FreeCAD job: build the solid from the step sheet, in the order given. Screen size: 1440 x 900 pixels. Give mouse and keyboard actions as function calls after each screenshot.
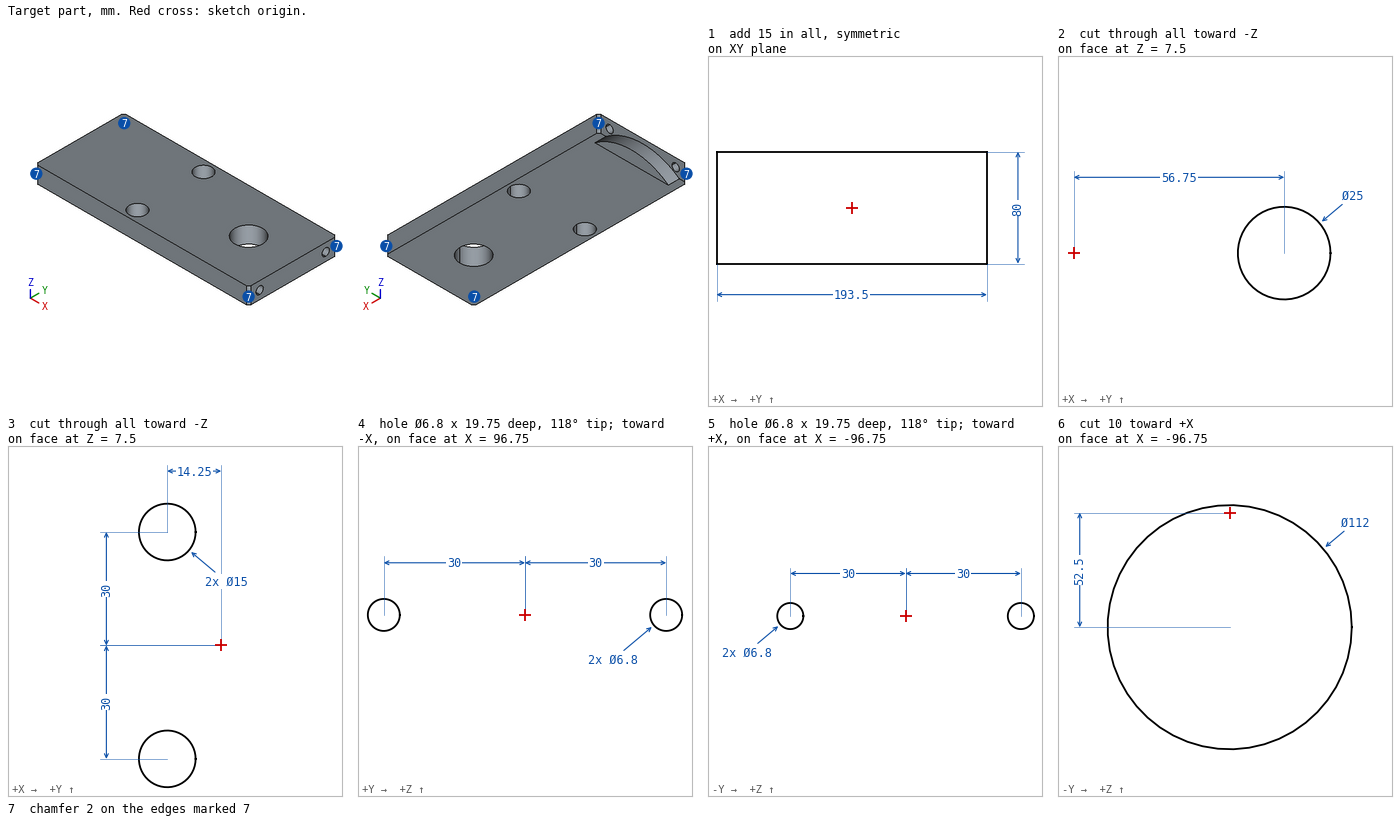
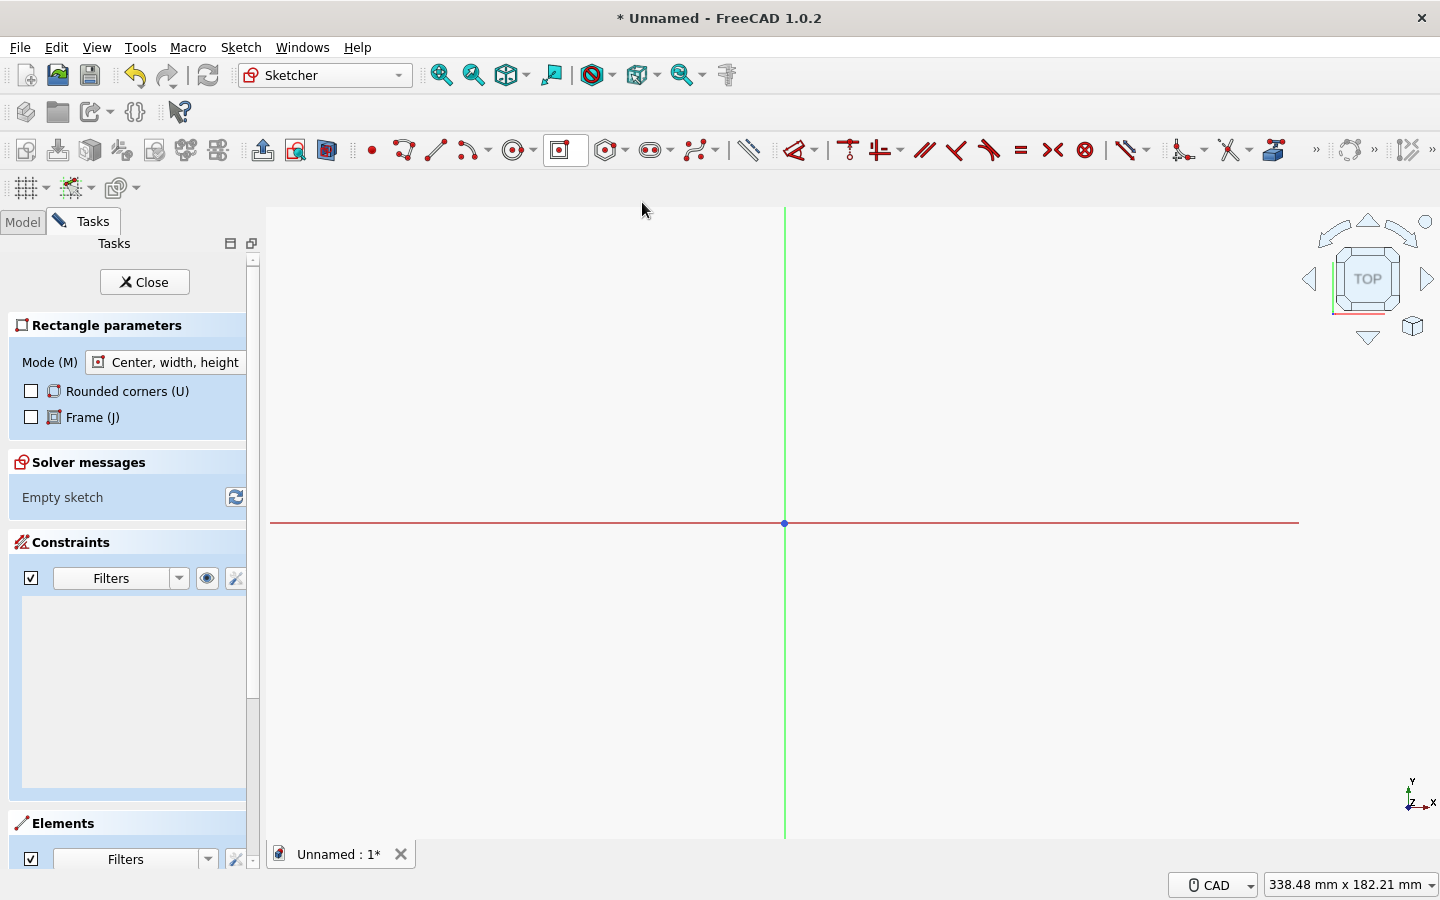
click(785, 523)
move(1120, 384)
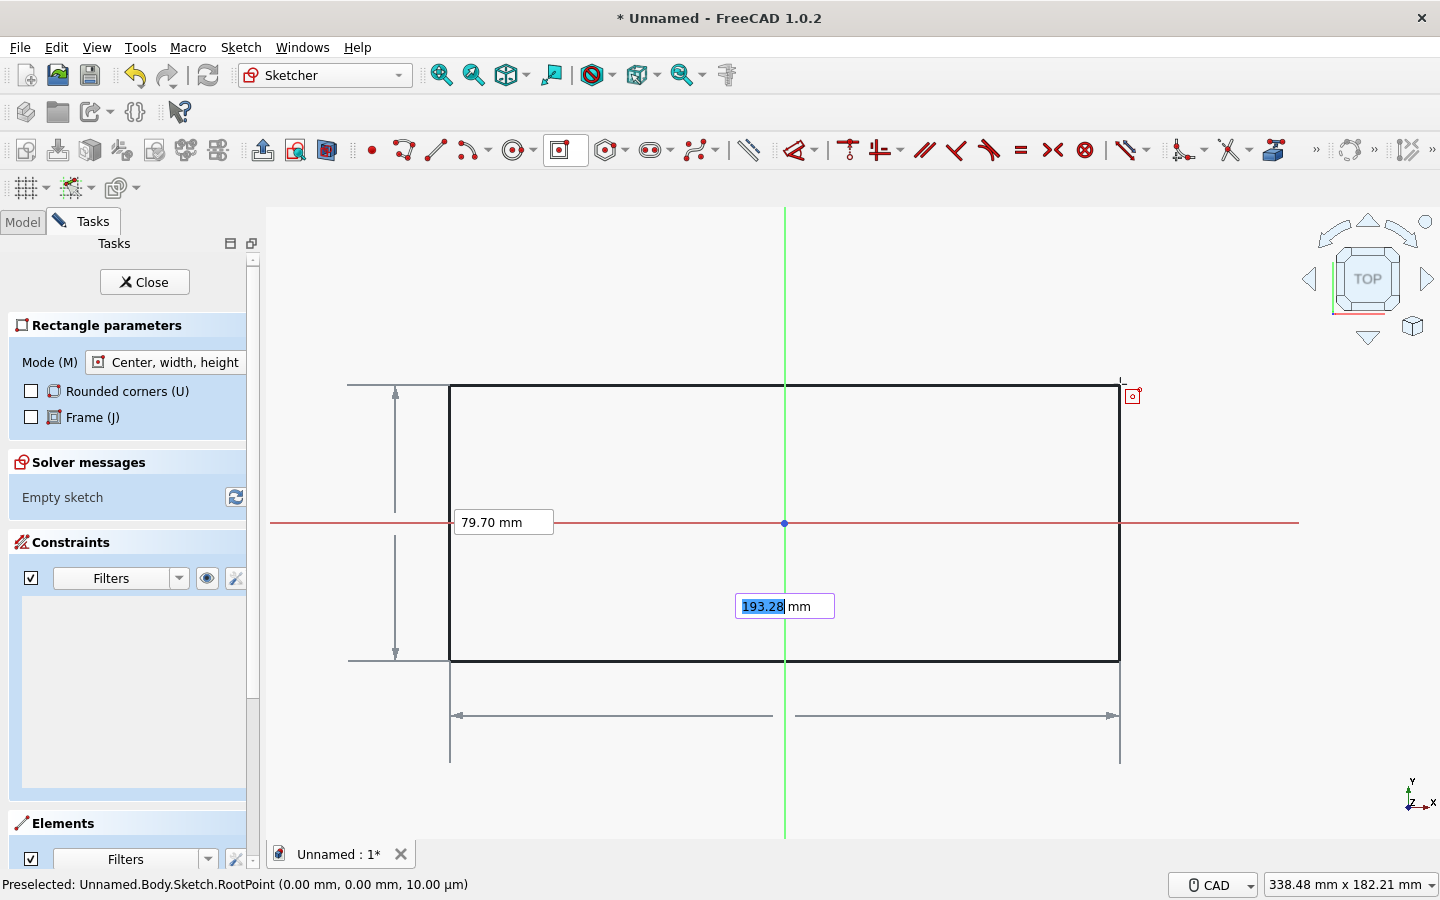
text(193.5)
key(Tab)
text(80)
key(Return)
key(Escape)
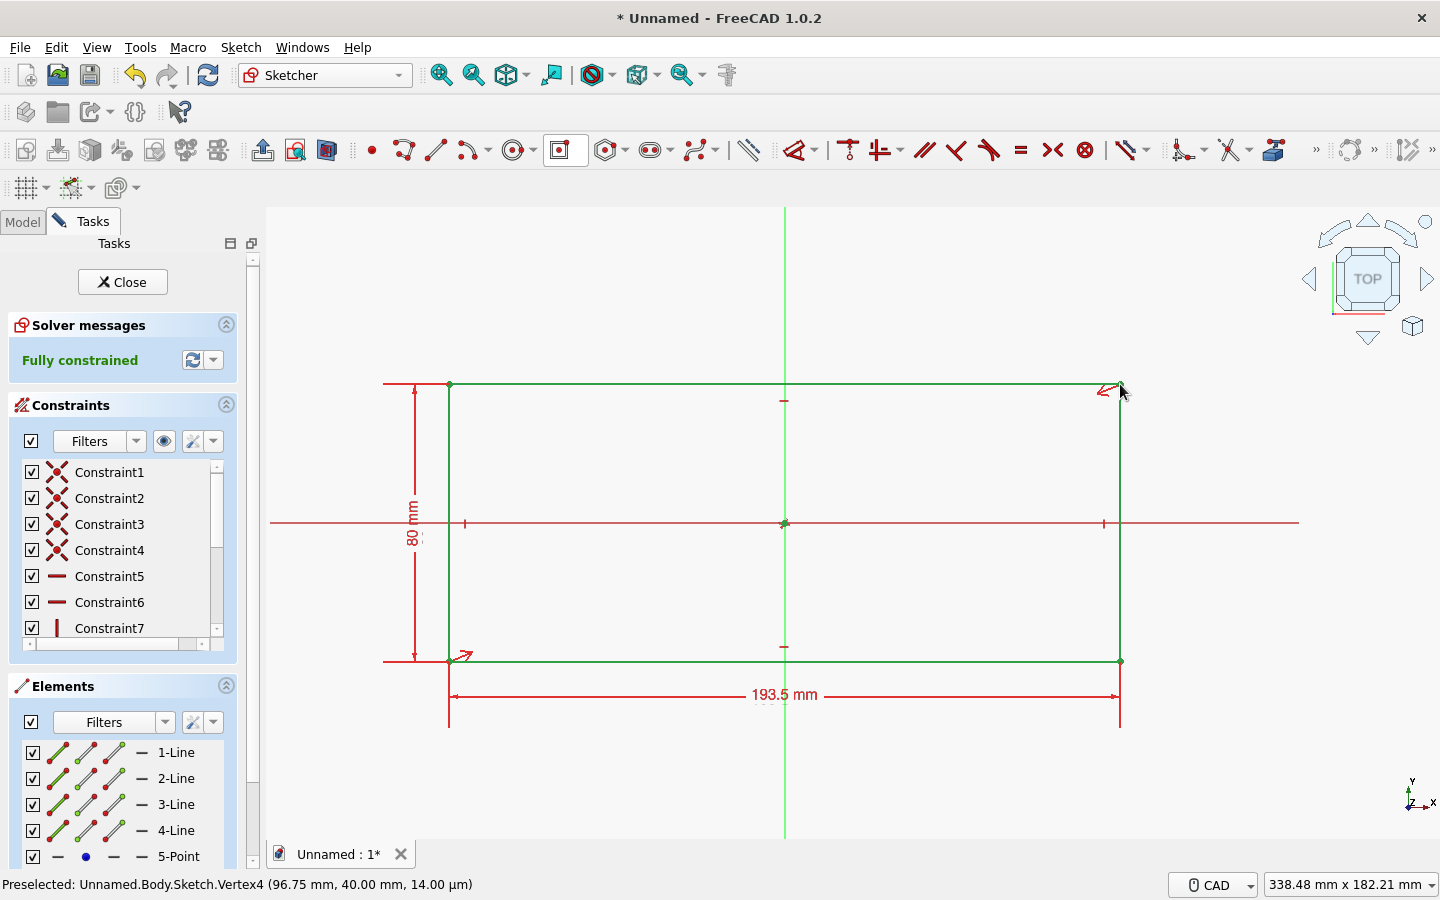
click(123, 282)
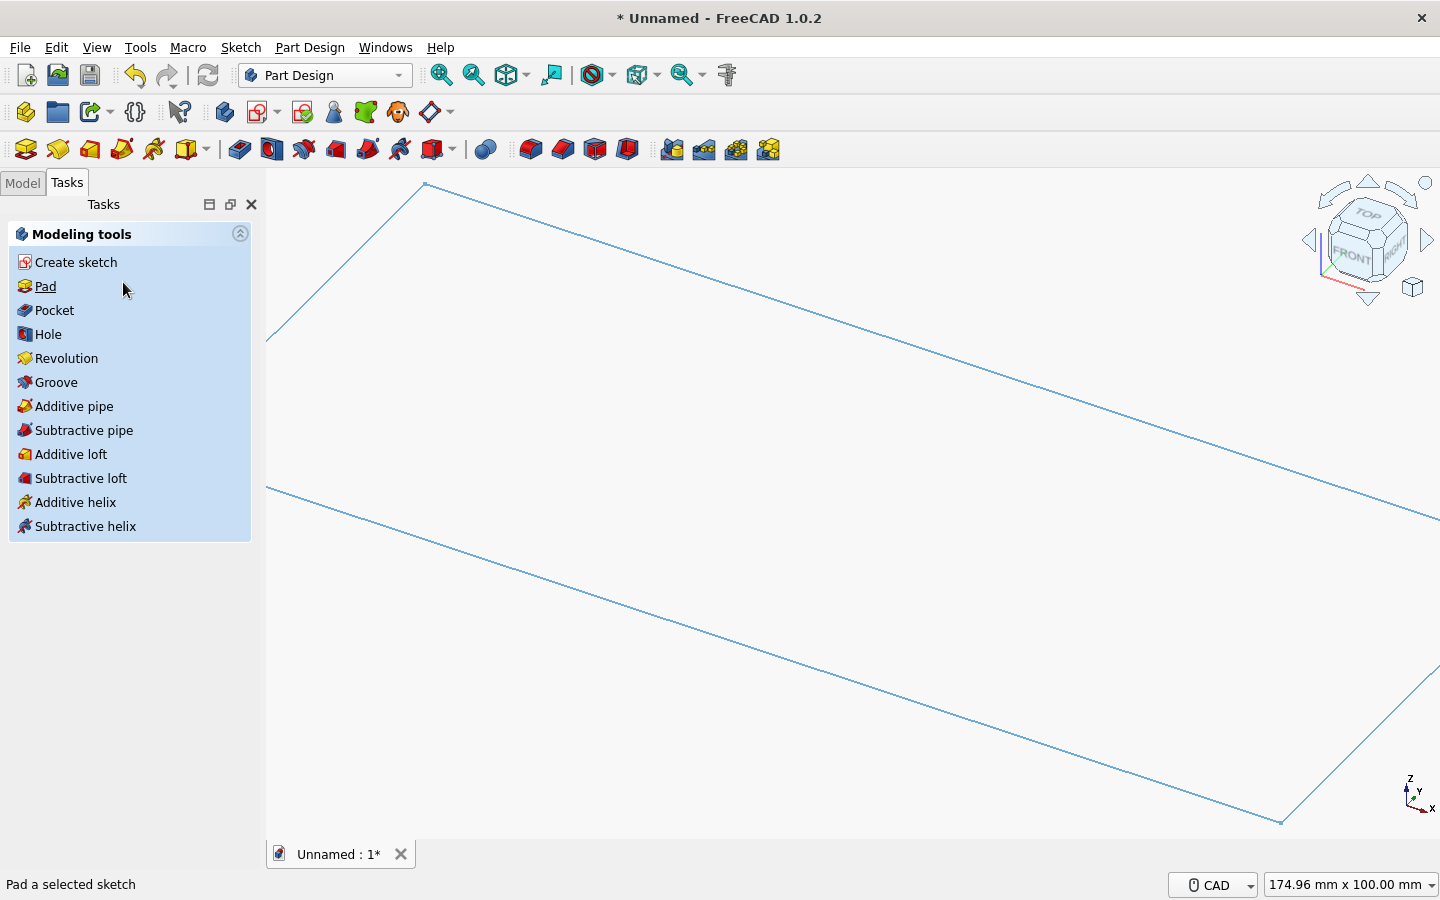
click(26, 150)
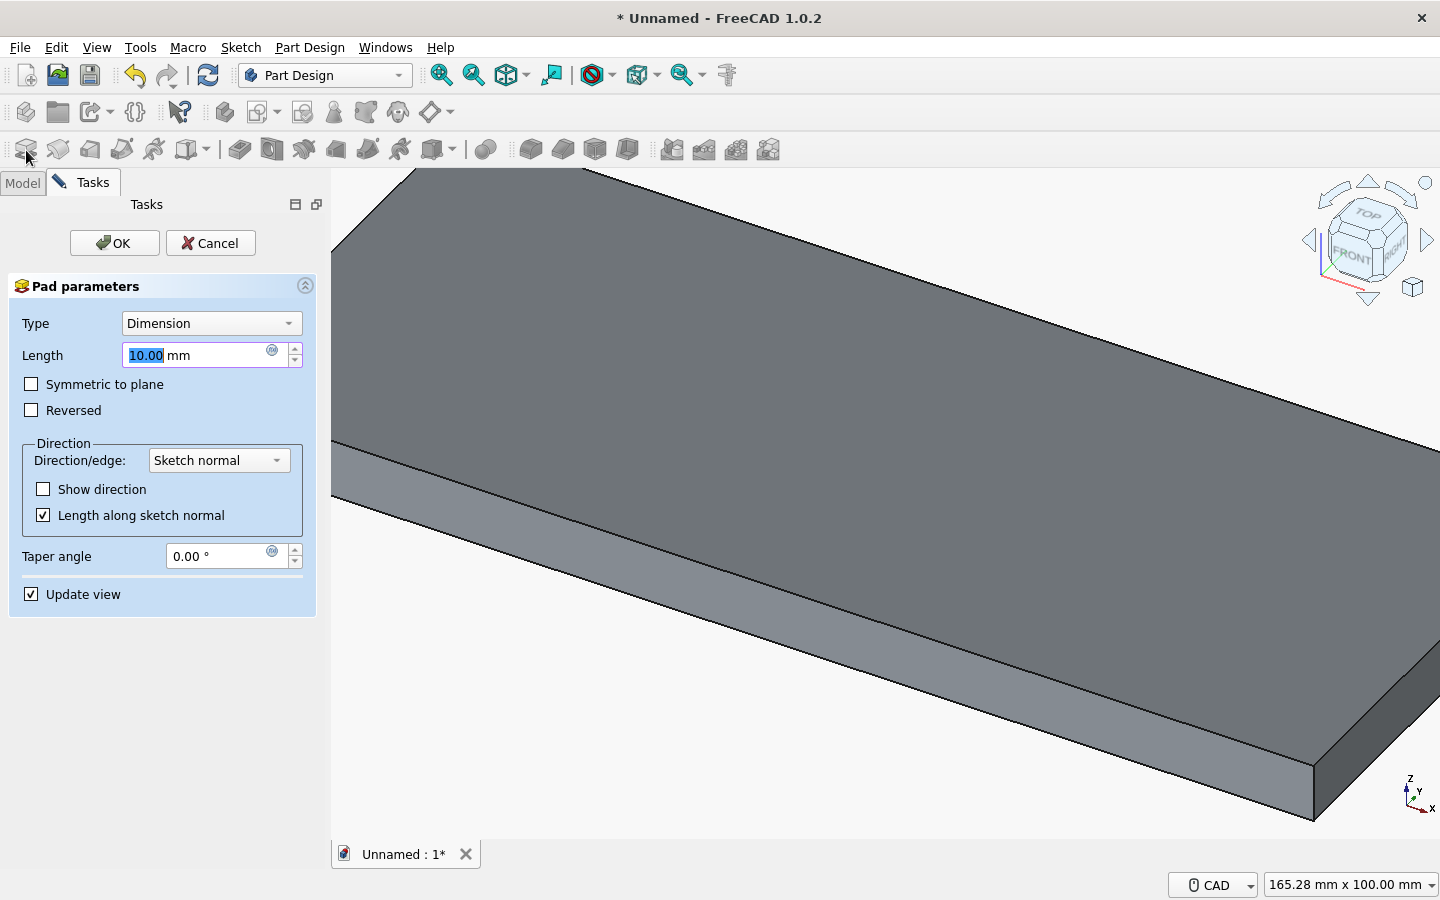
text(15)
key(Tab)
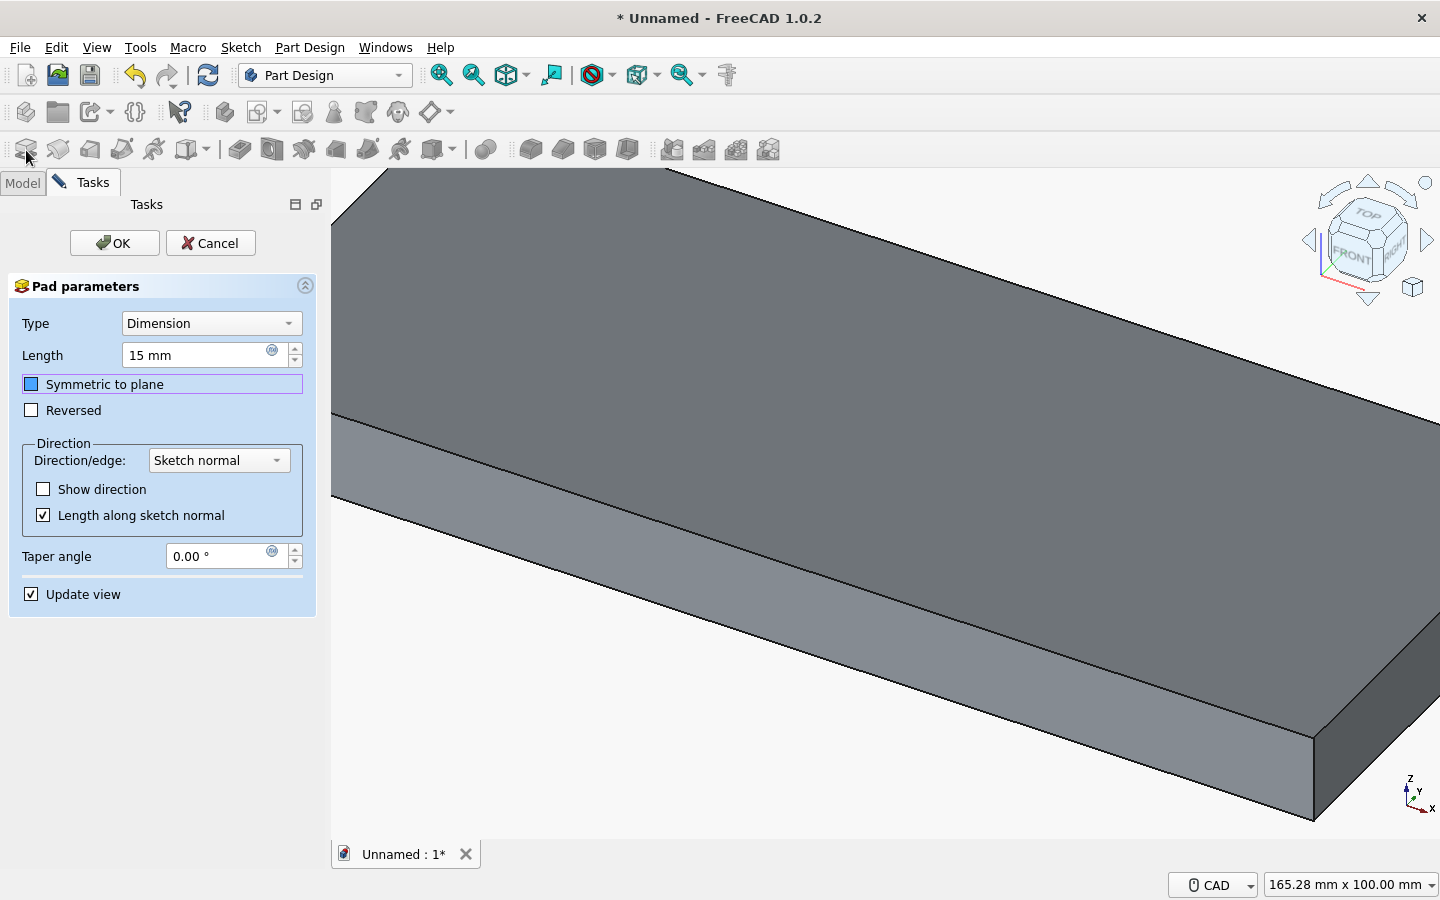
click(30, 384)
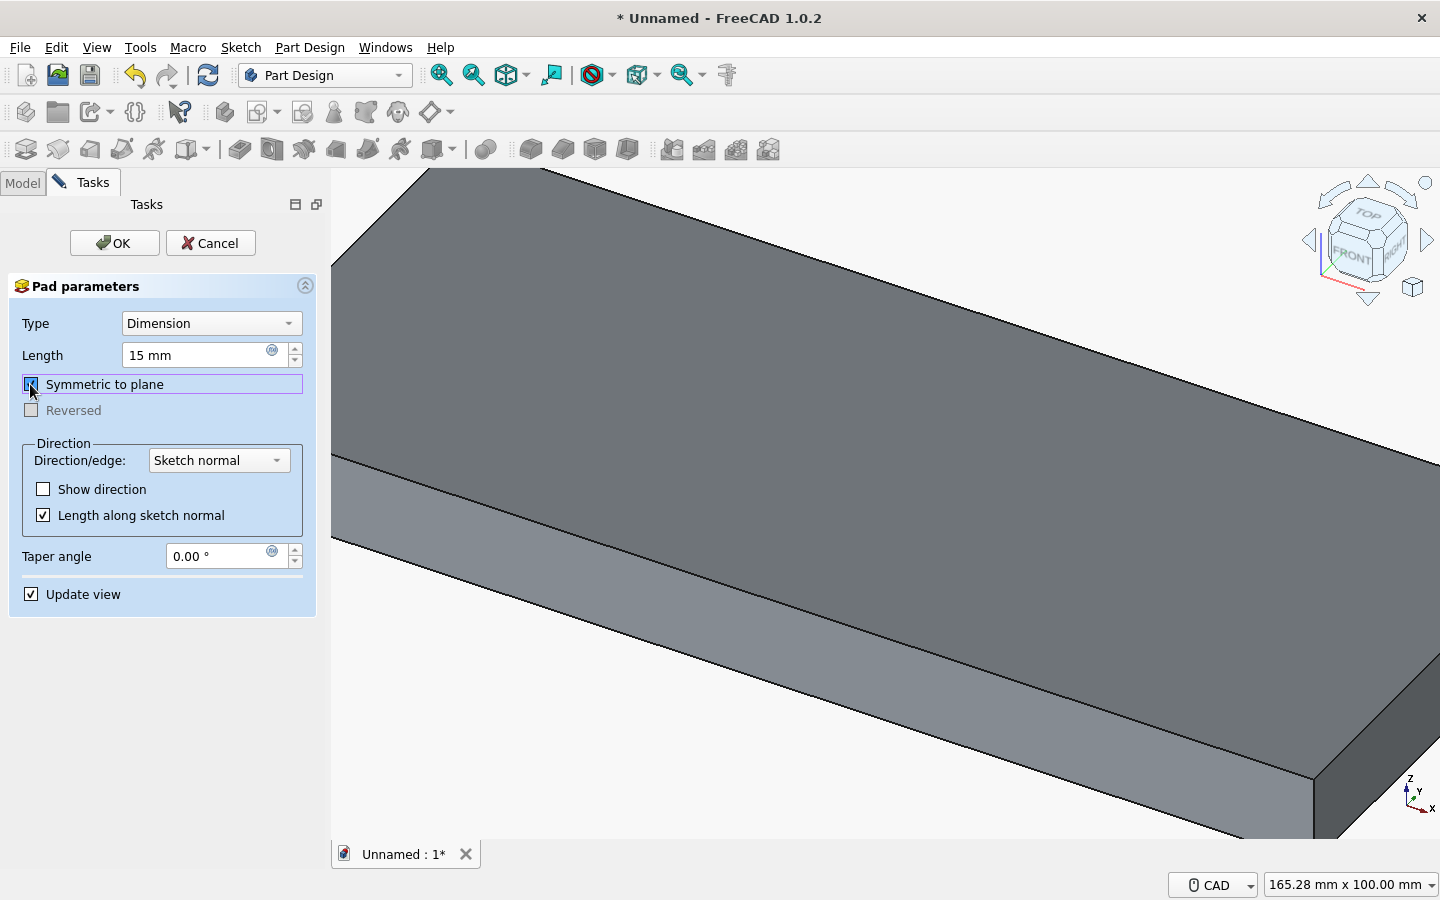
click(115, 243)